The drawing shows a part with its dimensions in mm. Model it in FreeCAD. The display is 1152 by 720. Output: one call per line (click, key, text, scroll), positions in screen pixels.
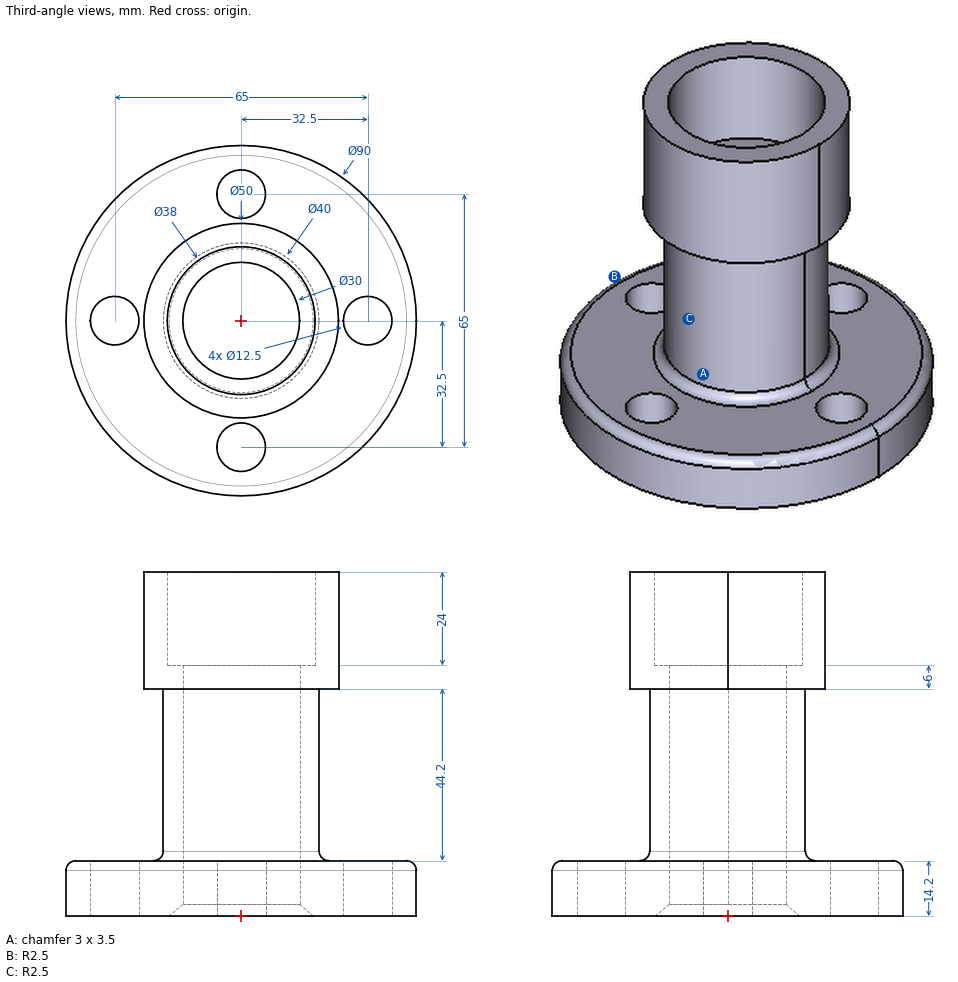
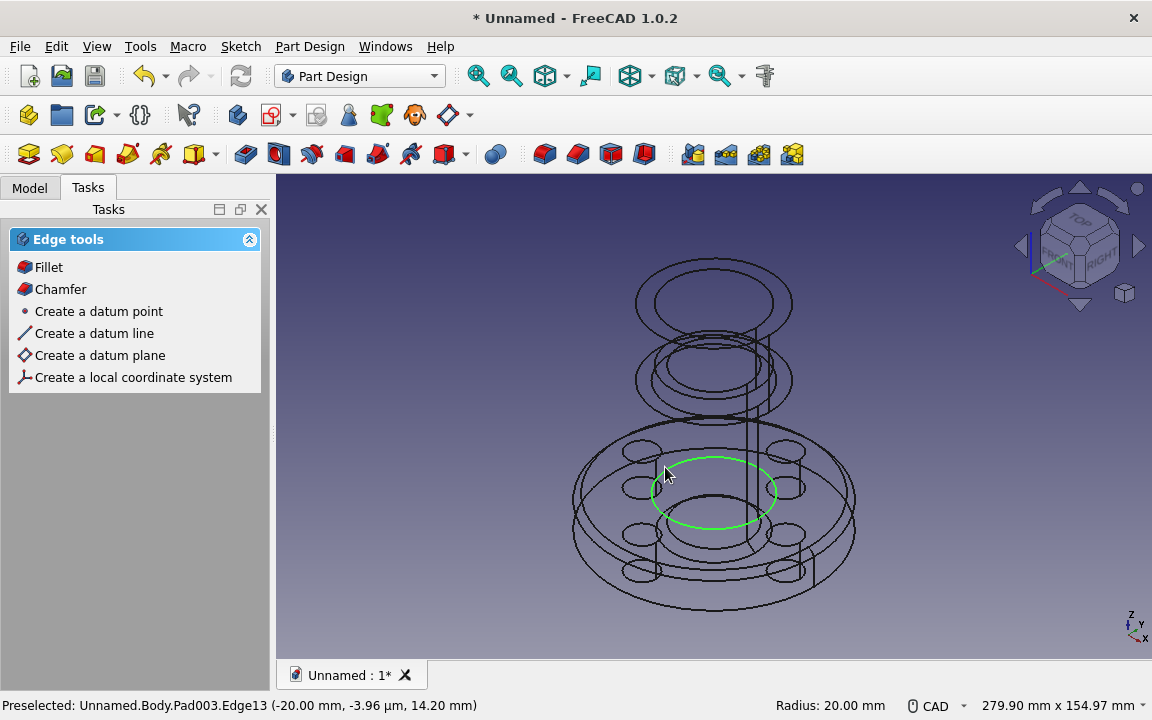
key(v)
key(1)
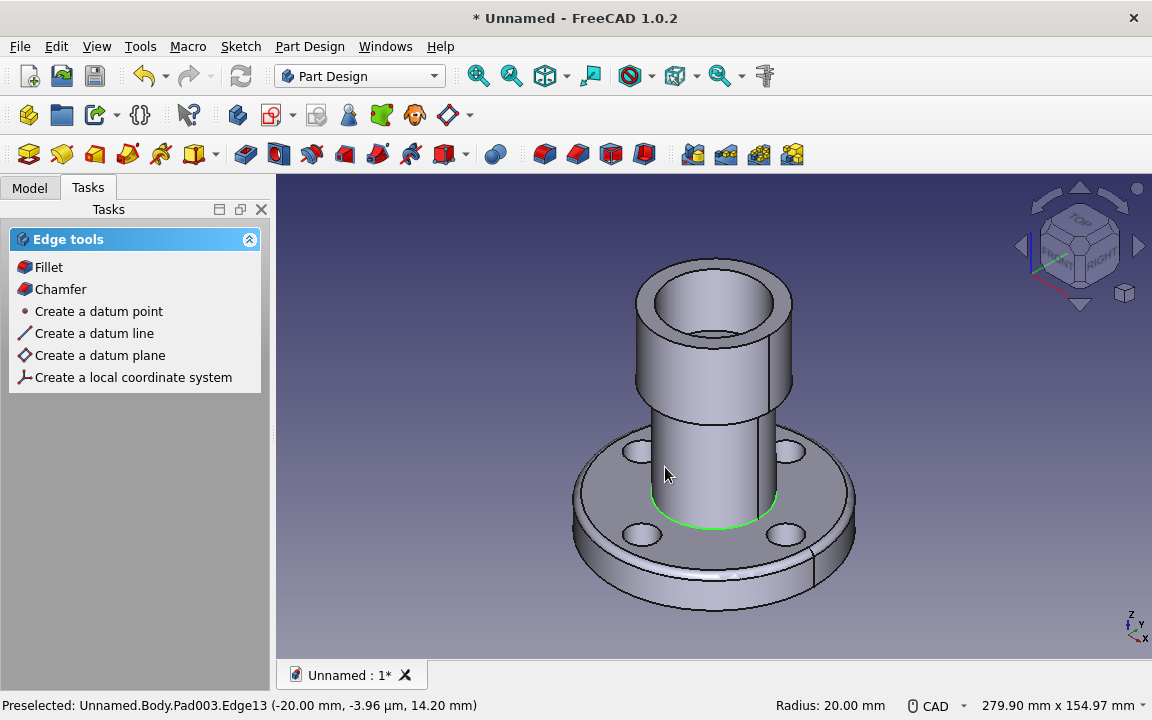
click(545, 154)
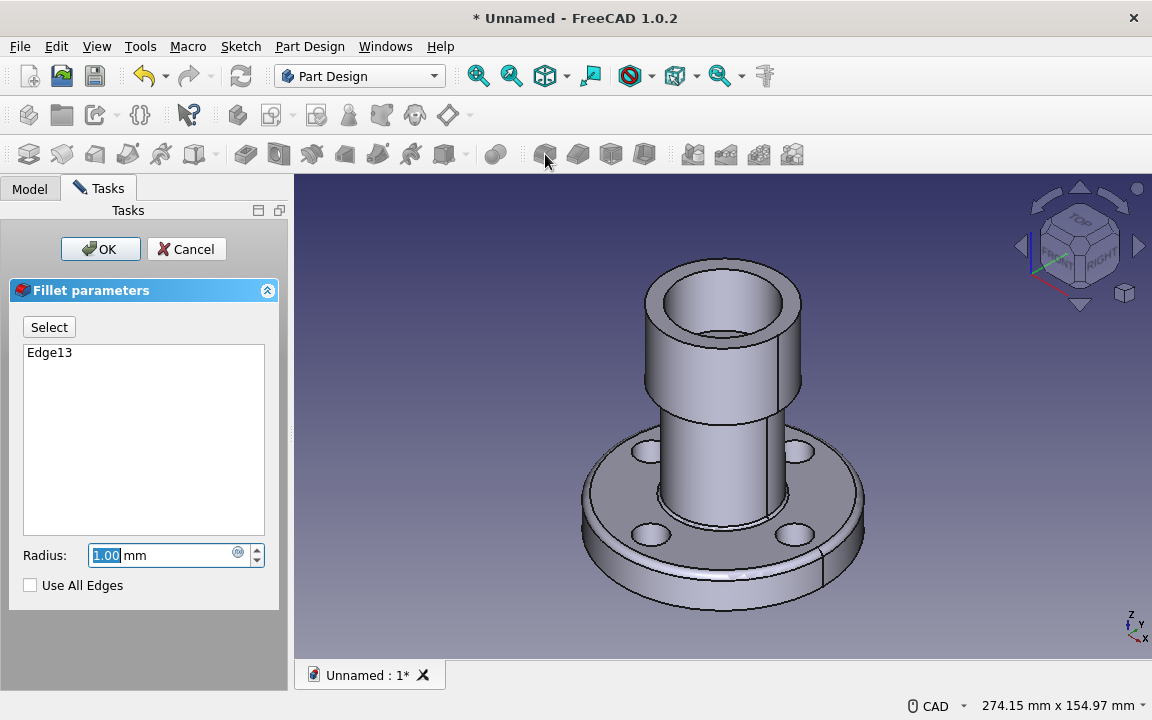
text(2.5)
key(Tab)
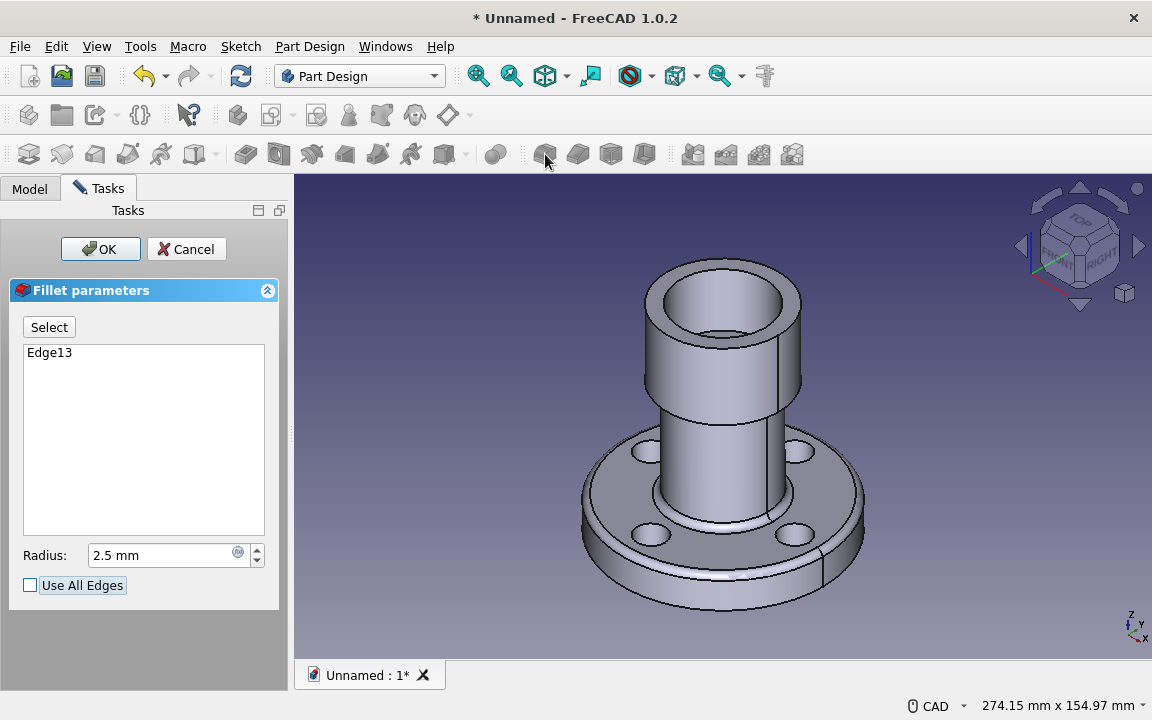
click(101, 249)